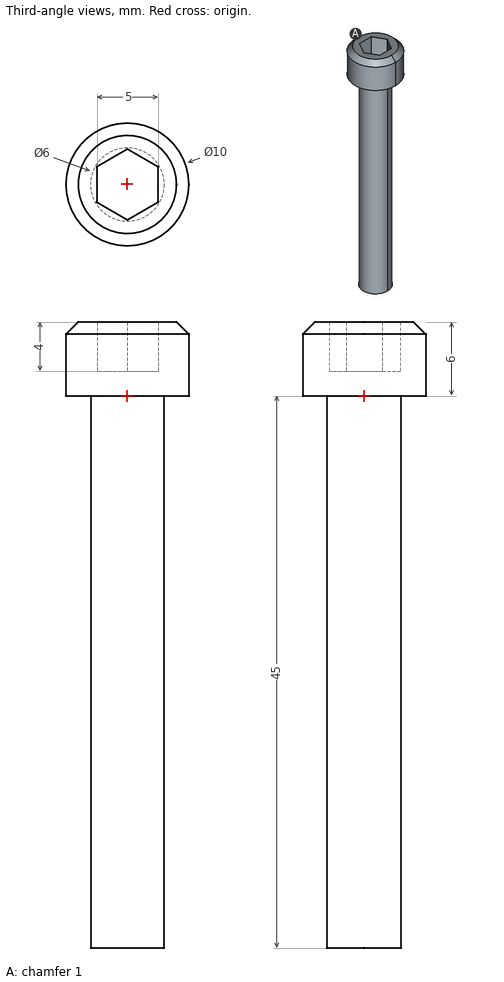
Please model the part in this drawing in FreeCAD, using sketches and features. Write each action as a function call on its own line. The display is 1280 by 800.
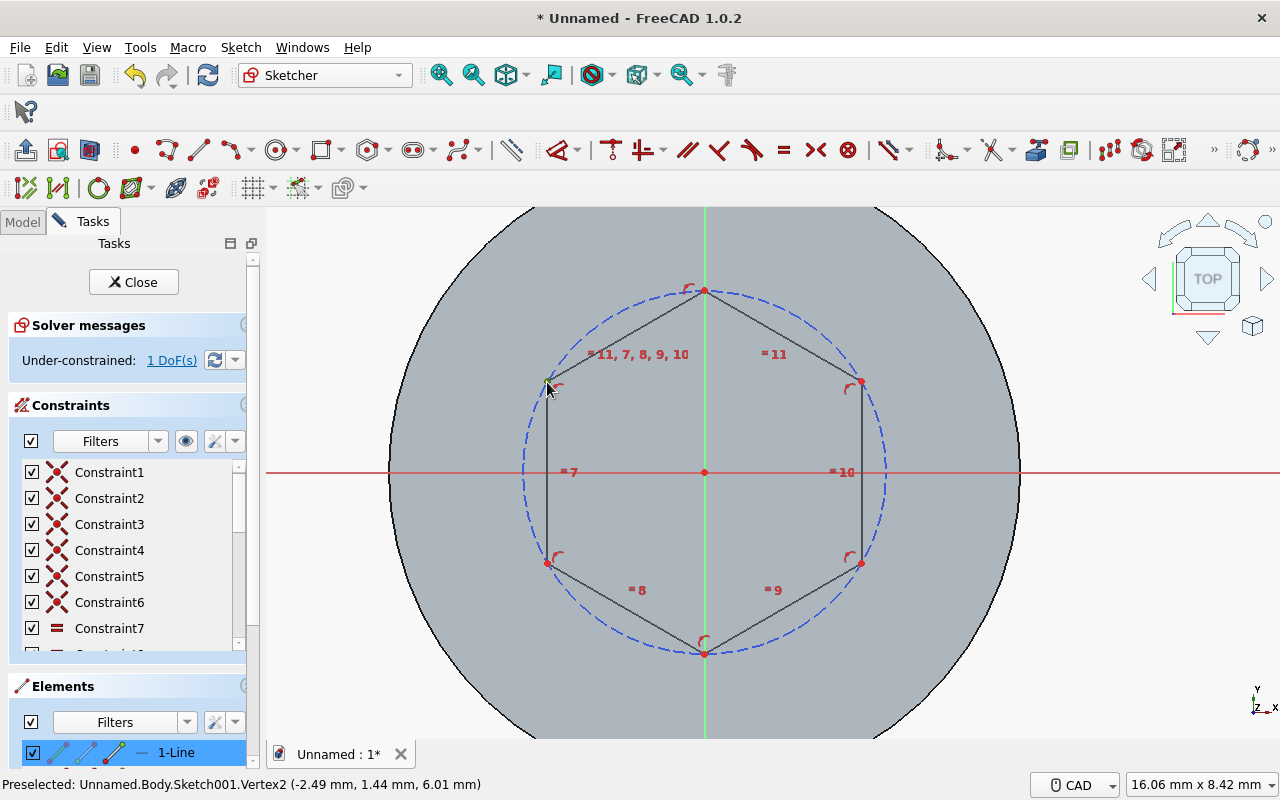
click(862, 563)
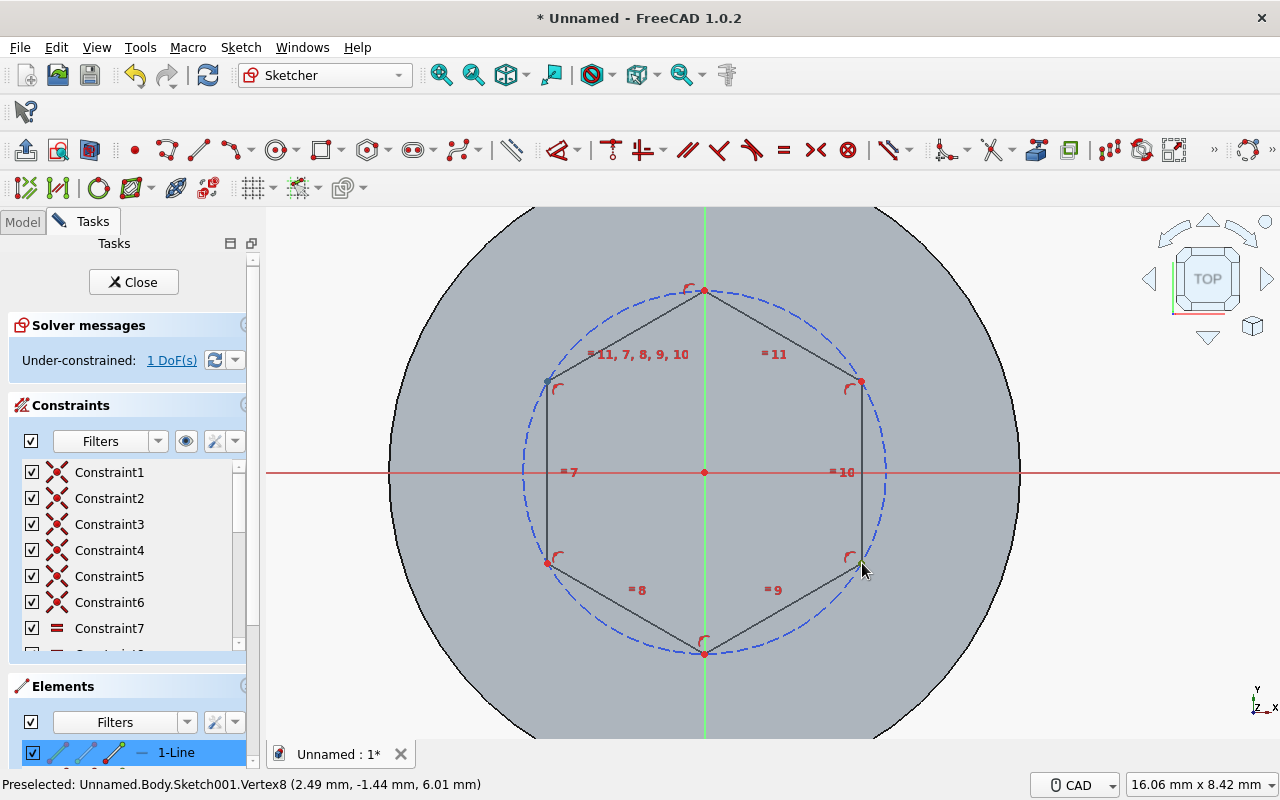
click(580, 150)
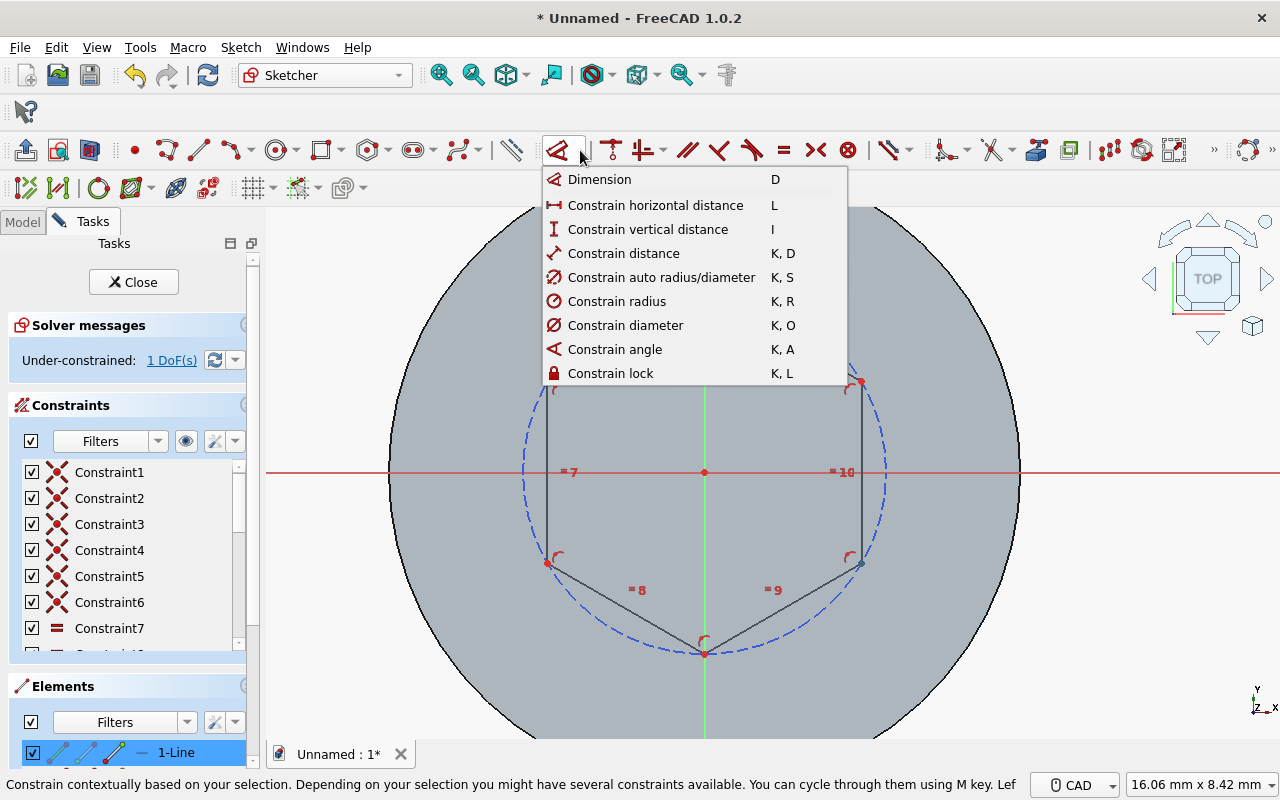
click(695, 205)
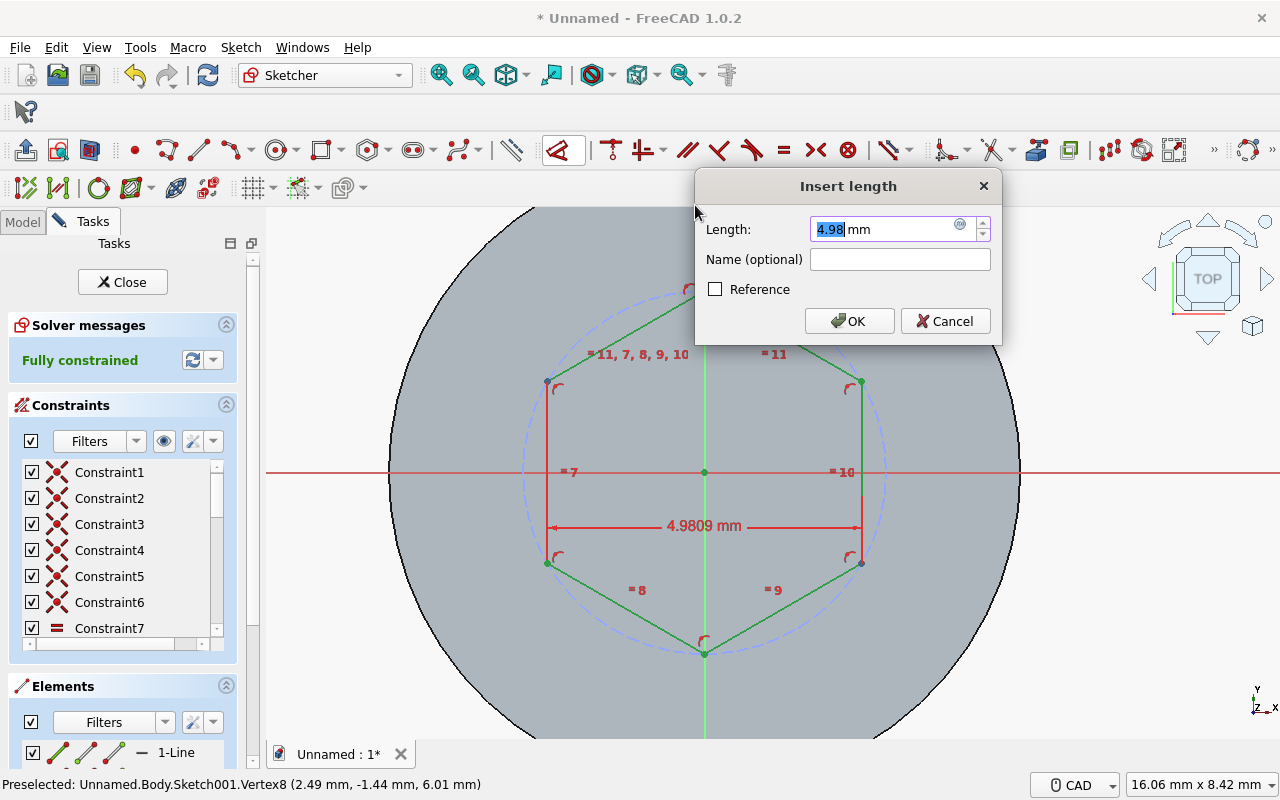
text(5)
key(Return)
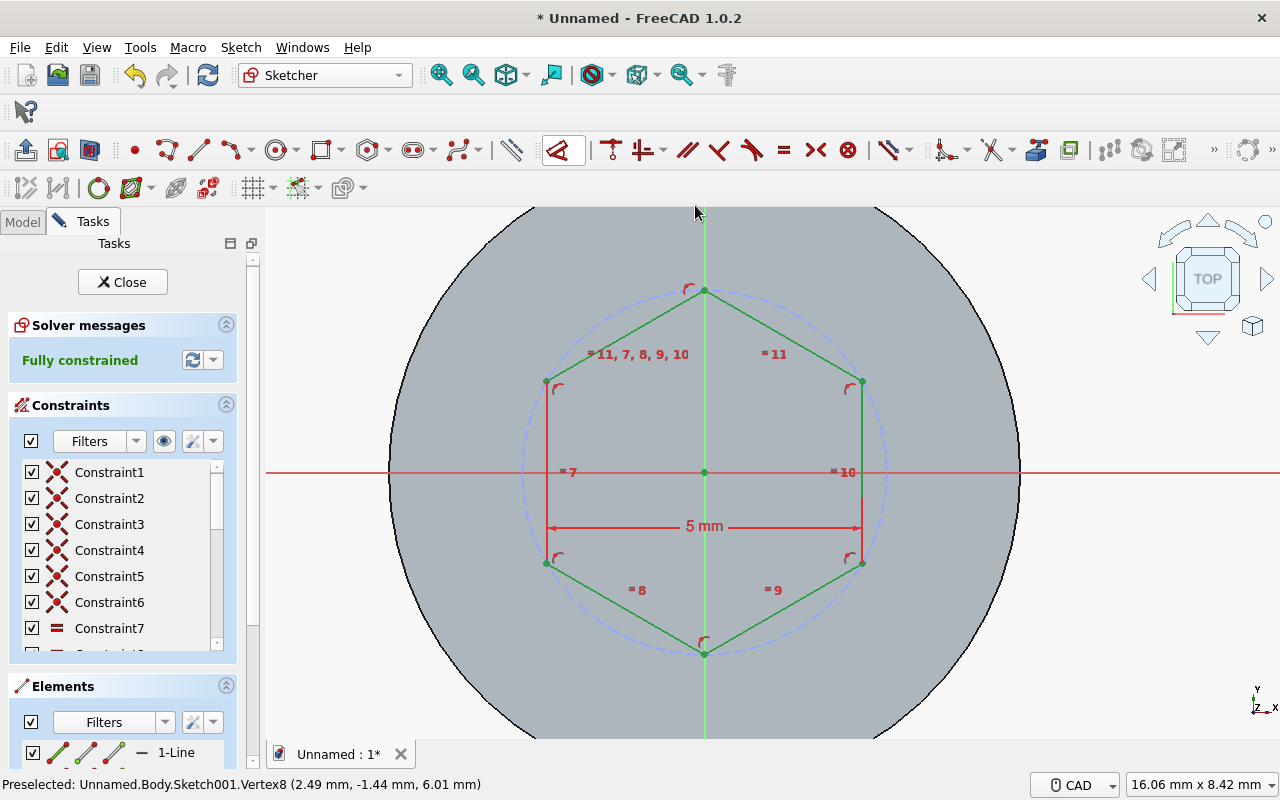
click(123, 282)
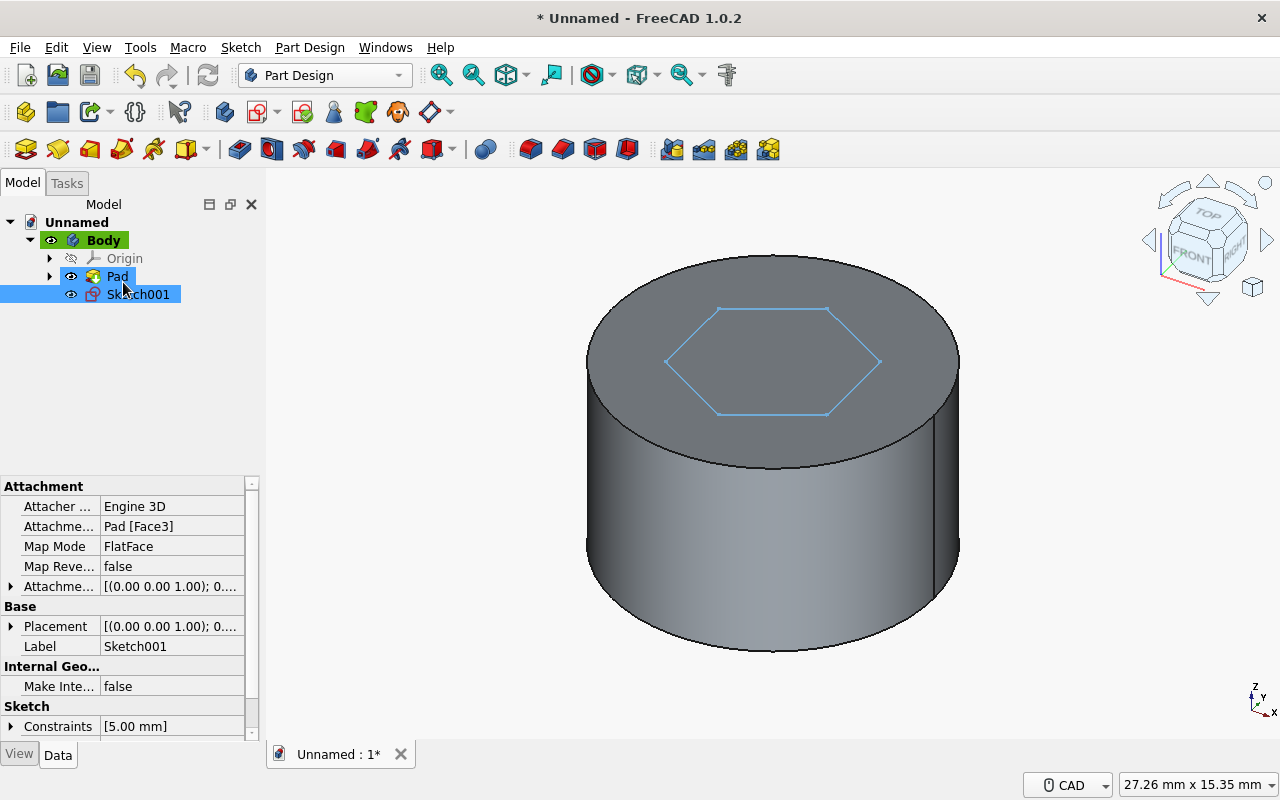
click(240, 150)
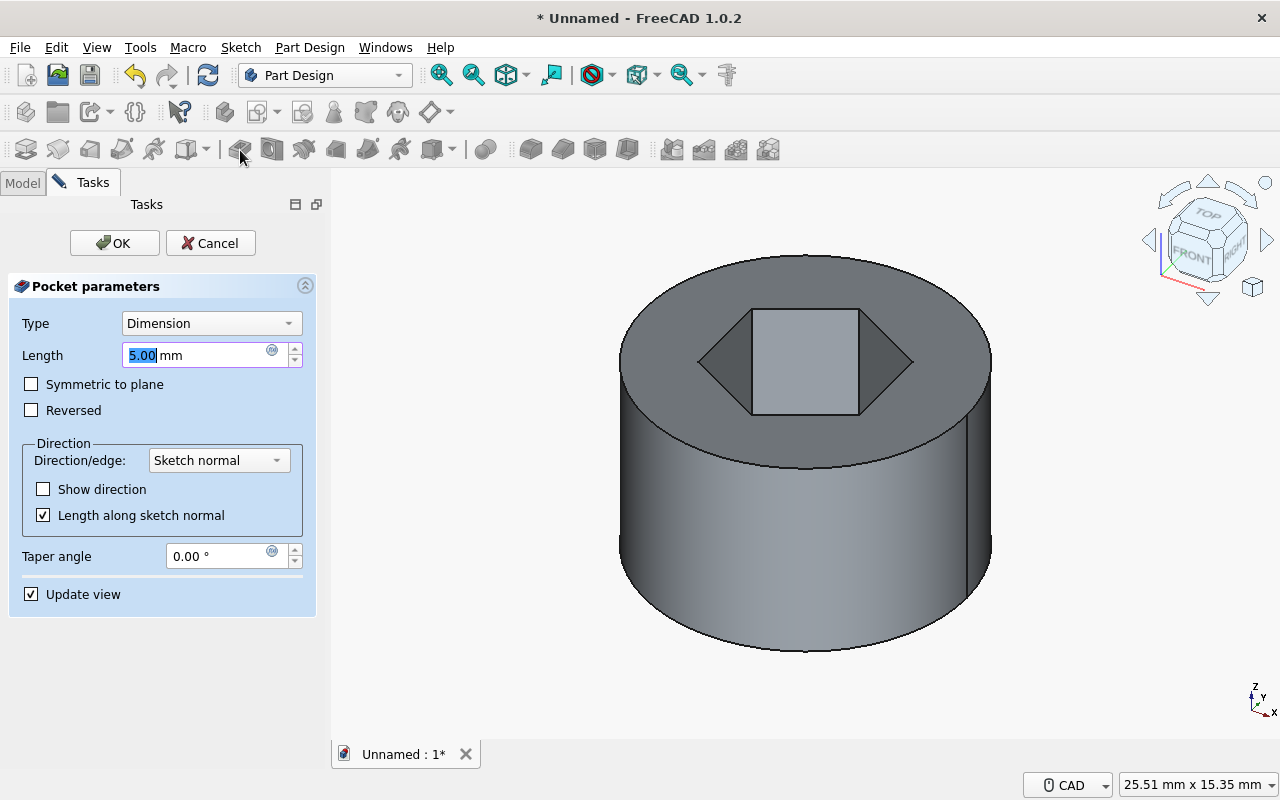
text(4)
key(Tab)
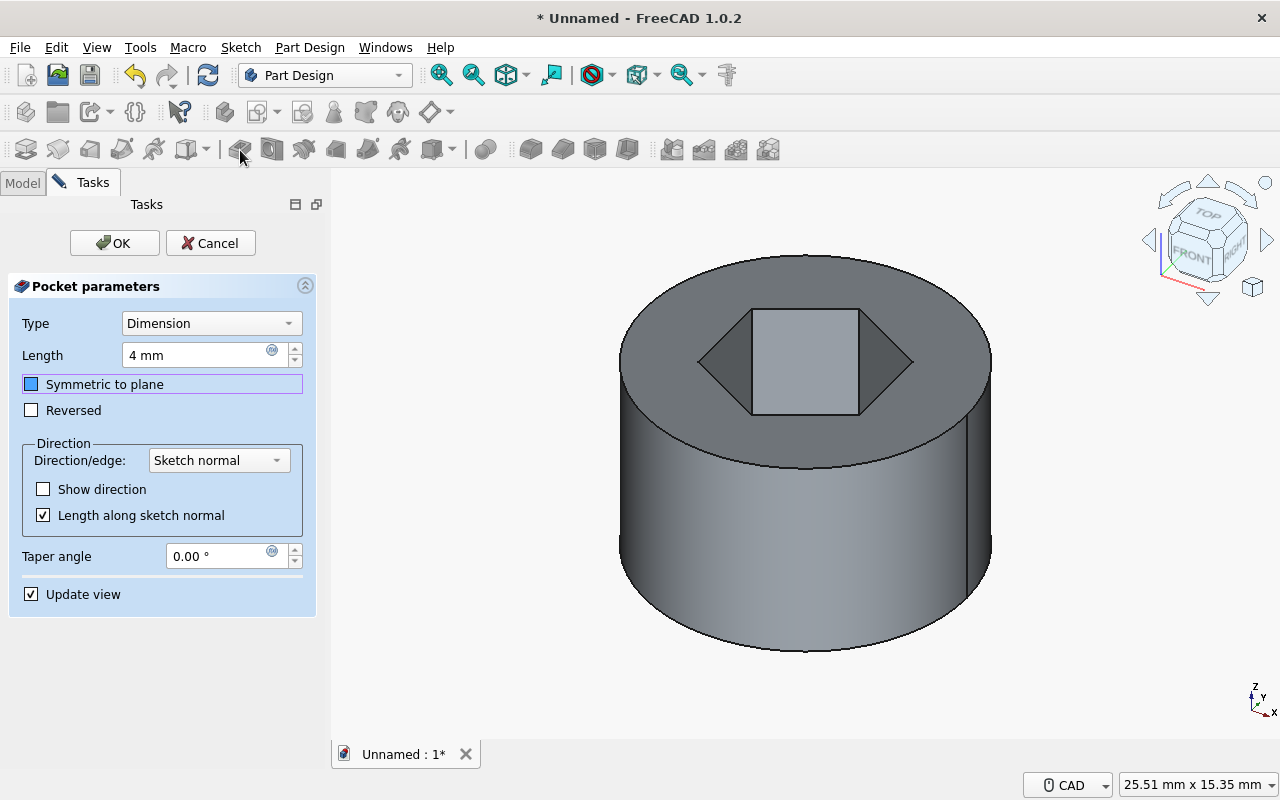
click(115, 243)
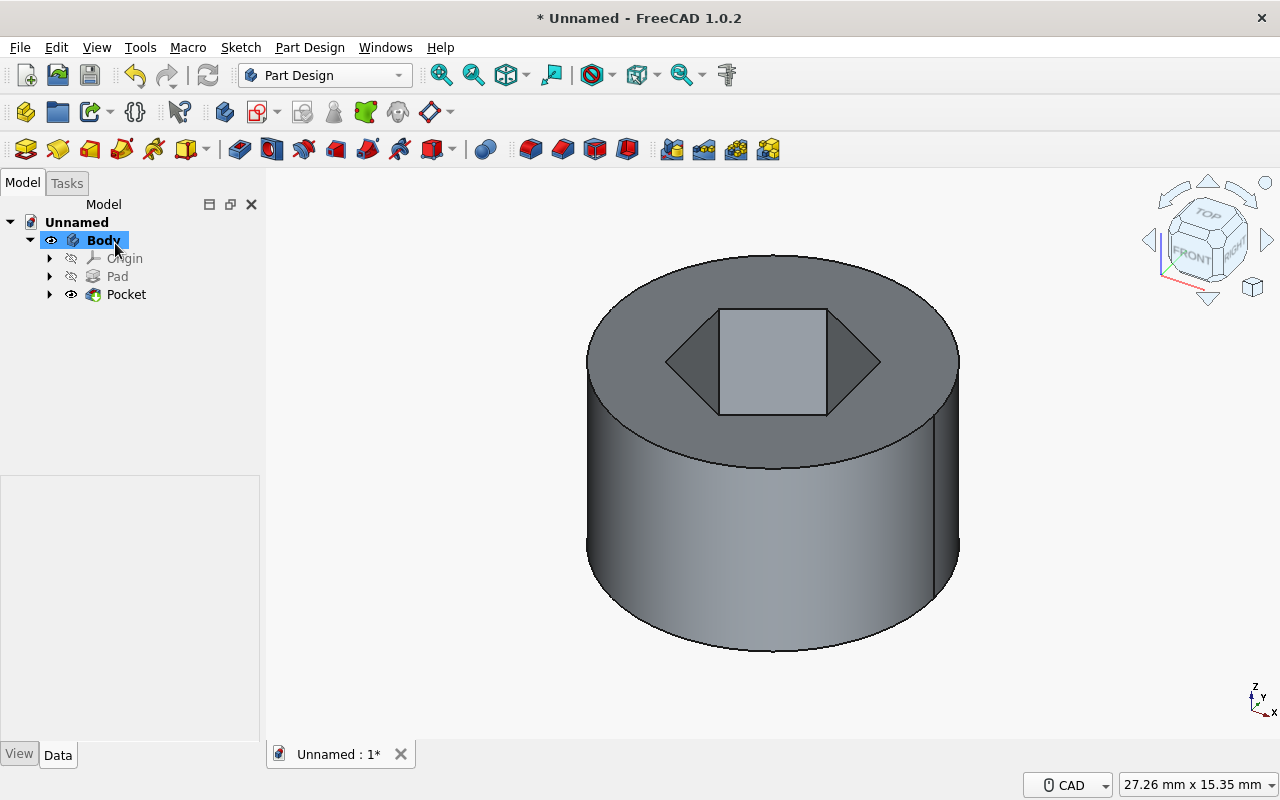
click(588, 372)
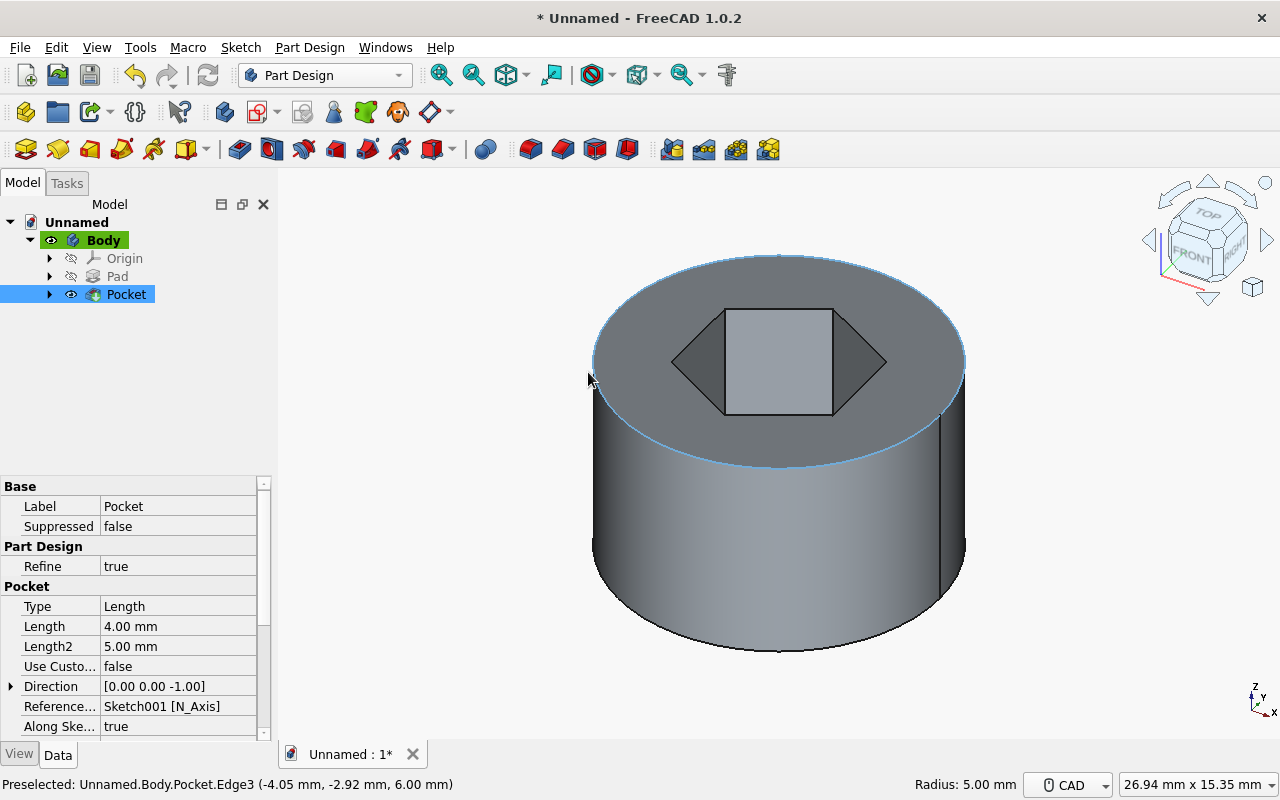
click(564, 150)